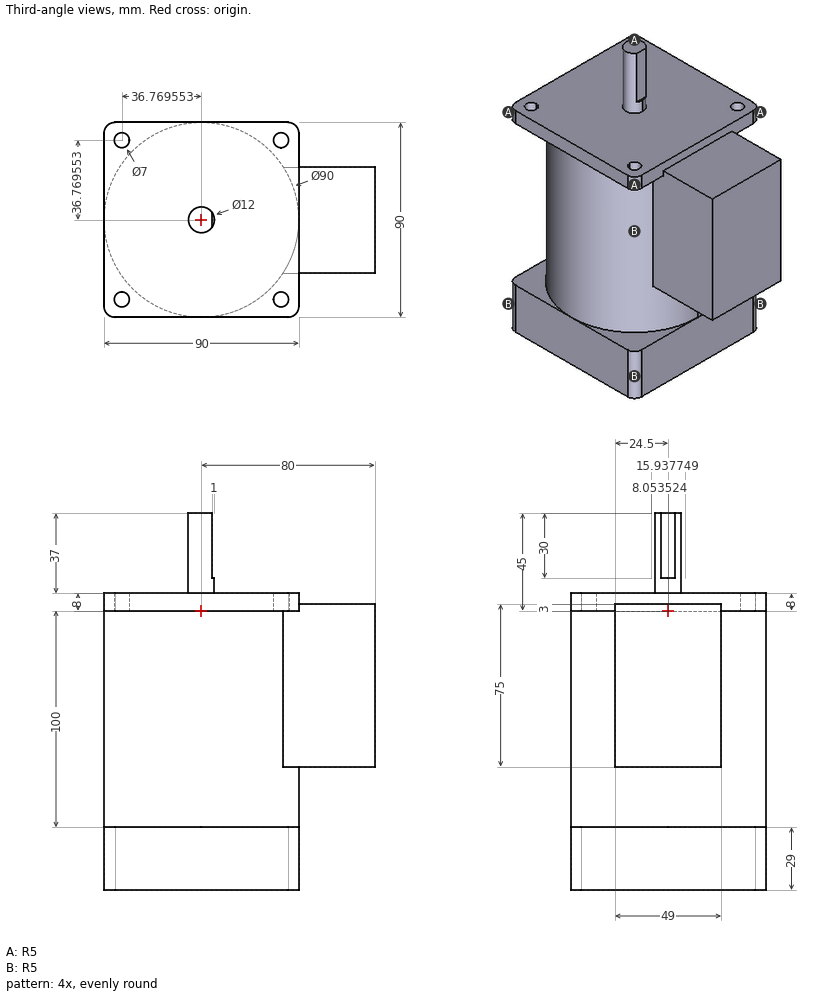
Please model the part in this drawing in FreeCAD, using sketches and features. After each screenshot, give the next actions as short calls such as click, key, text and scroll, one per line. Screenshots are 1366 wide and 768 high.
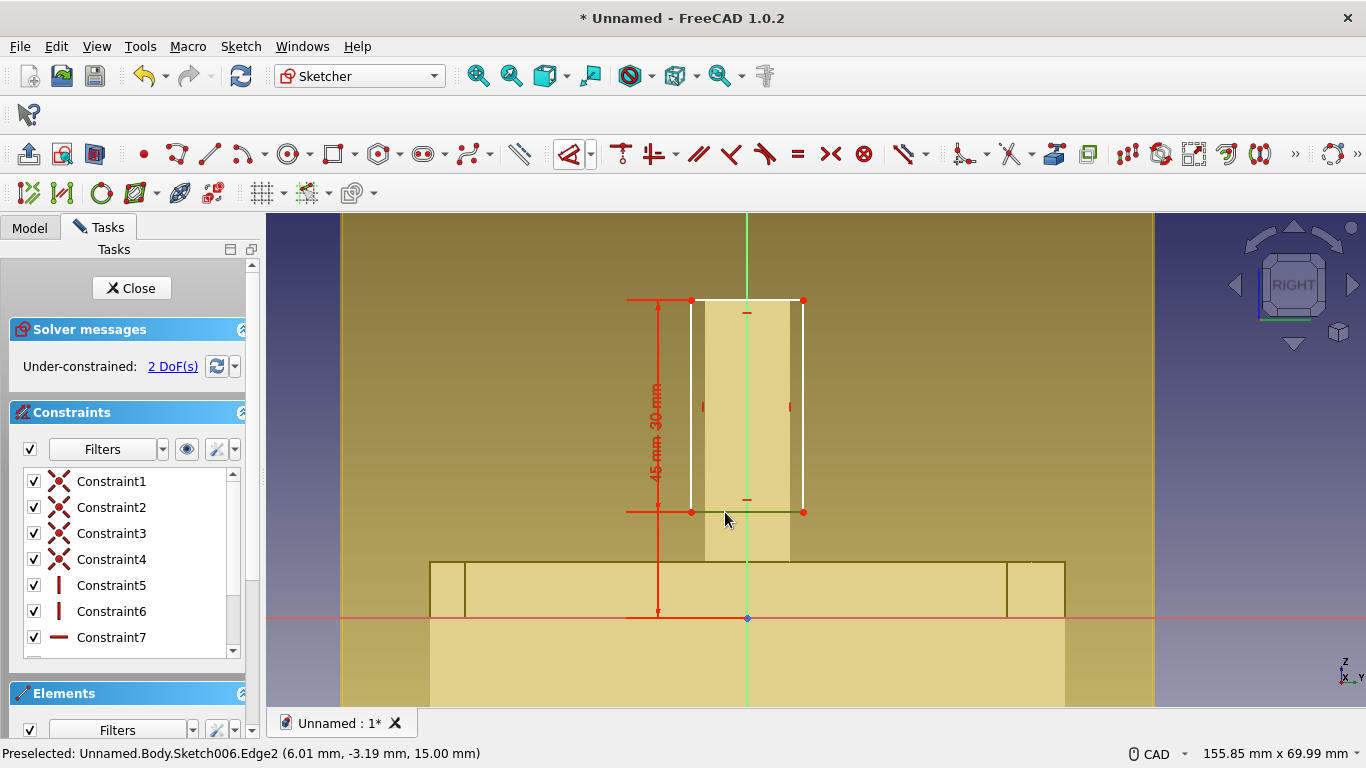
key(l)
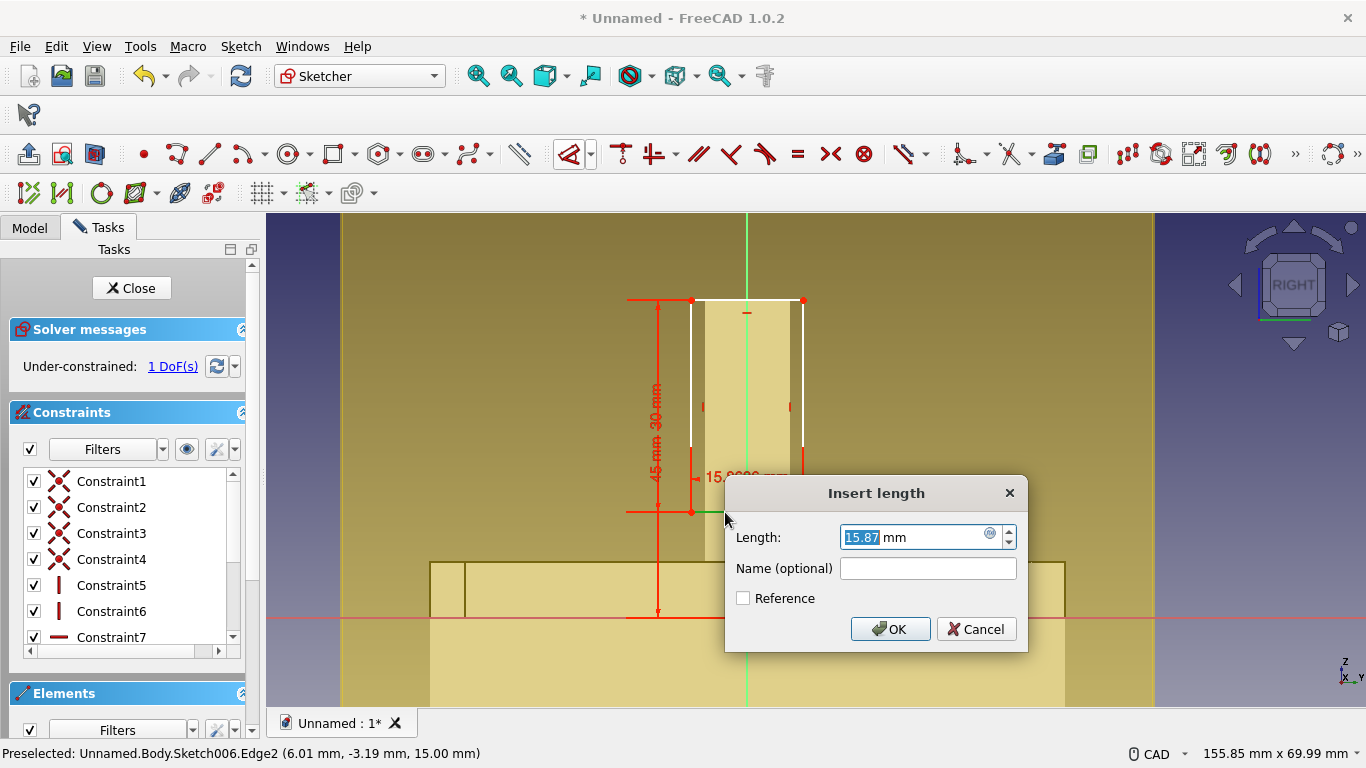
text(15.937749)
key(Return)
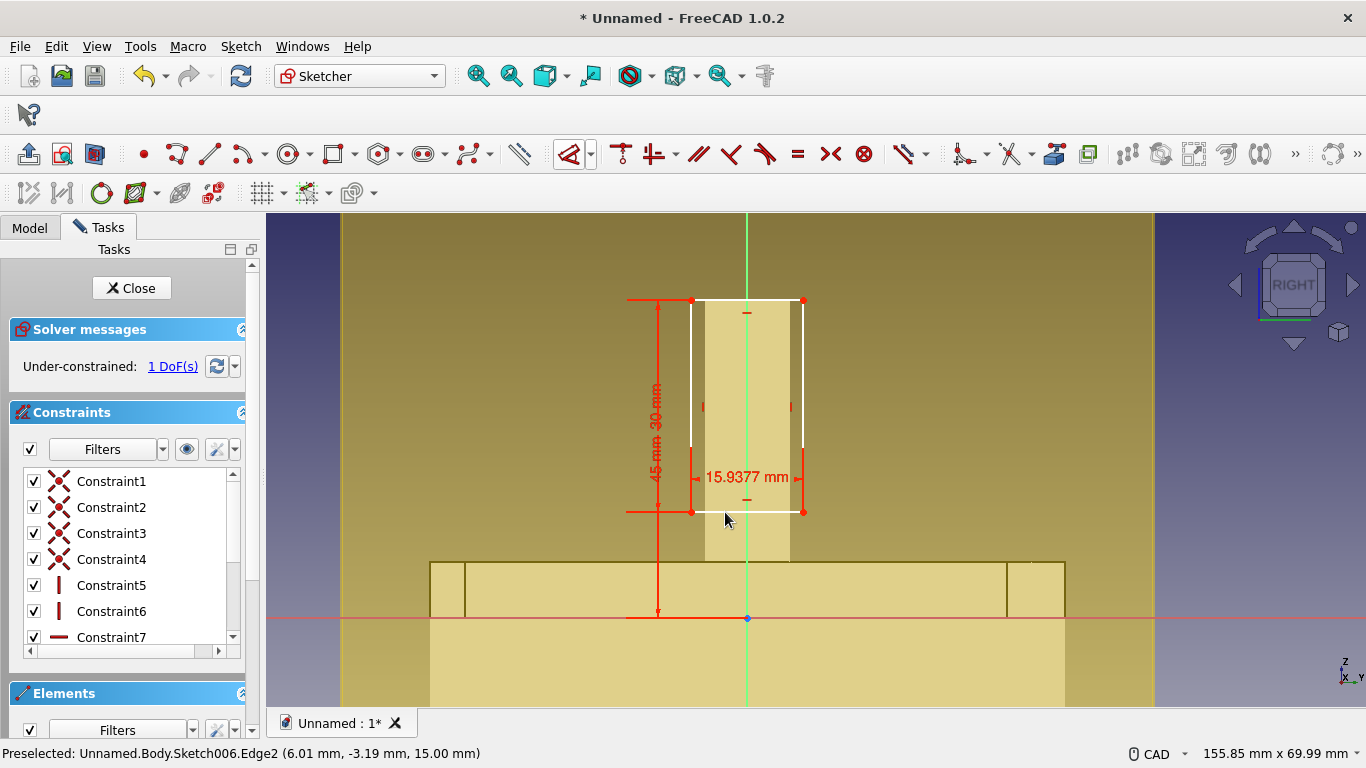
click(691, 300)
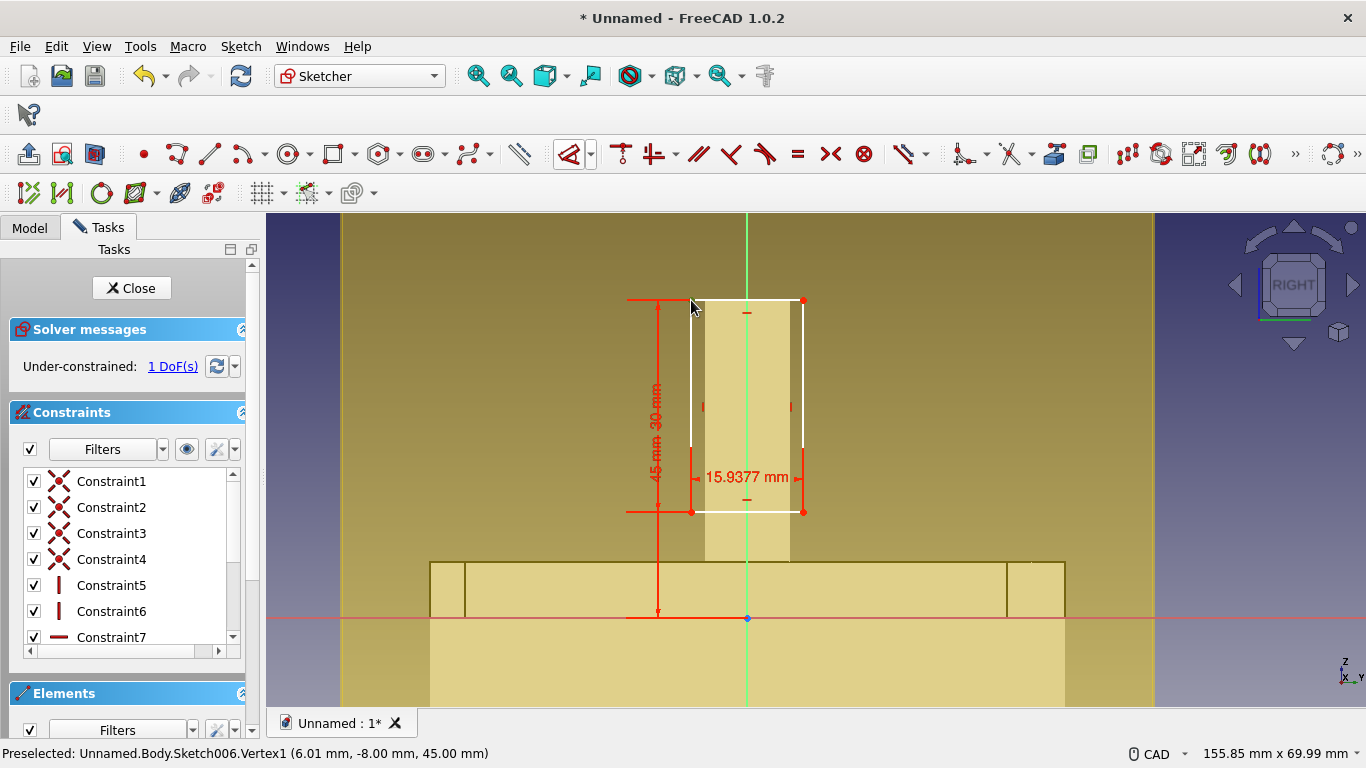
key(l)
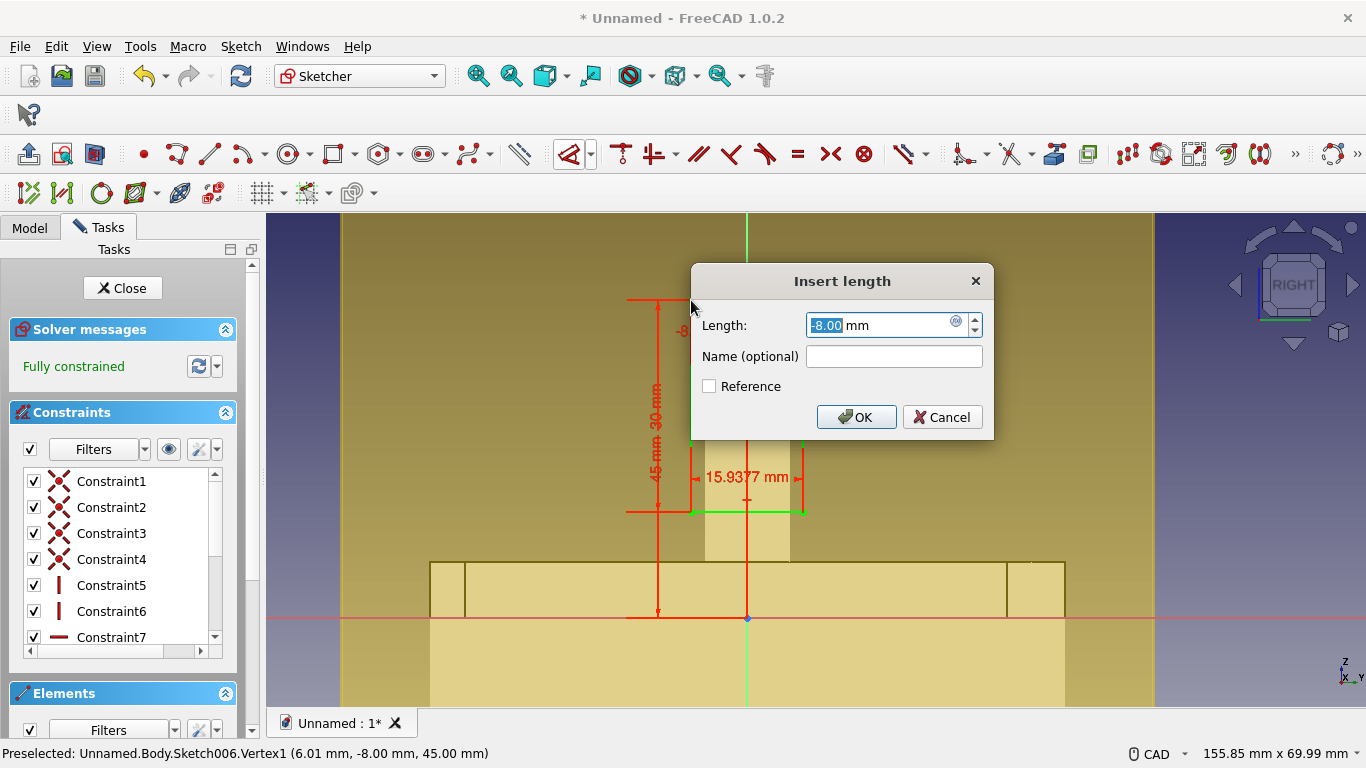
text(-8.053524)
key(Return)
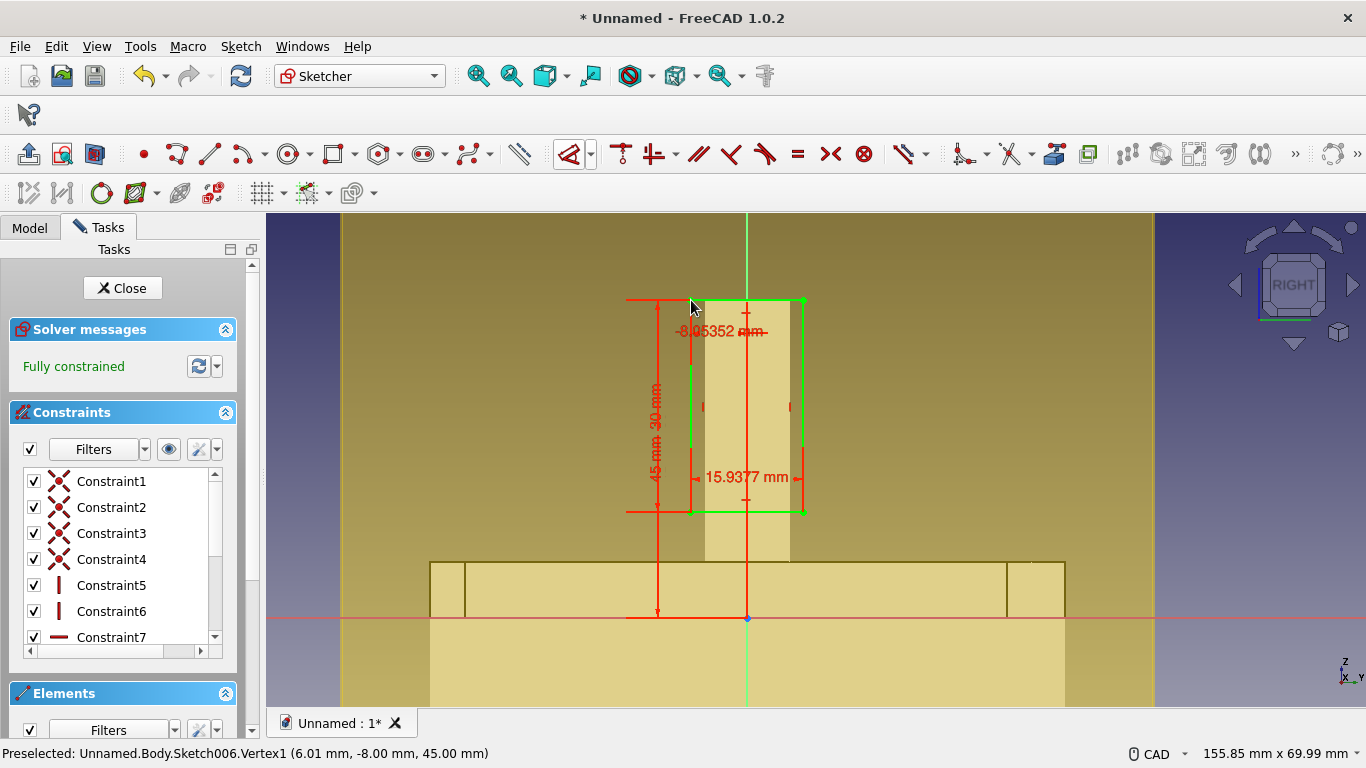
click(123, 288)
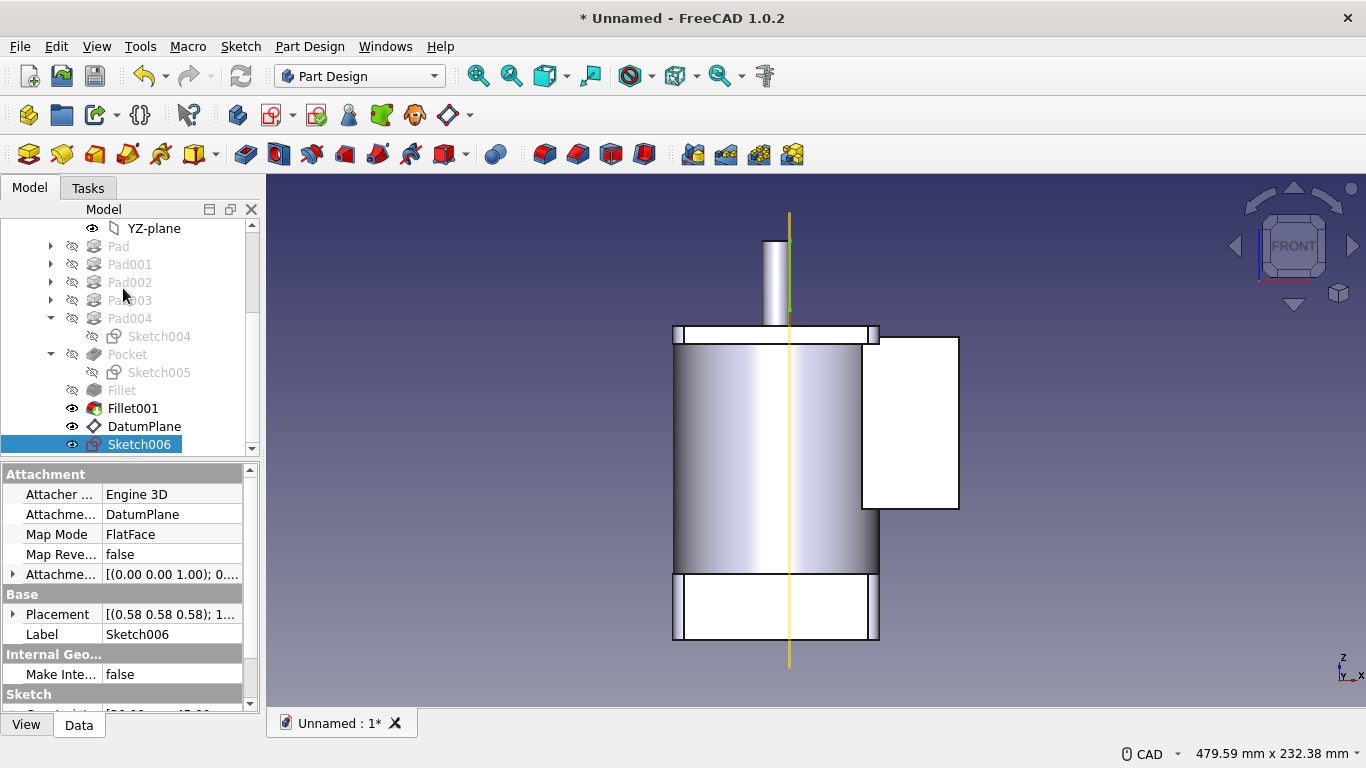
click(246, 154)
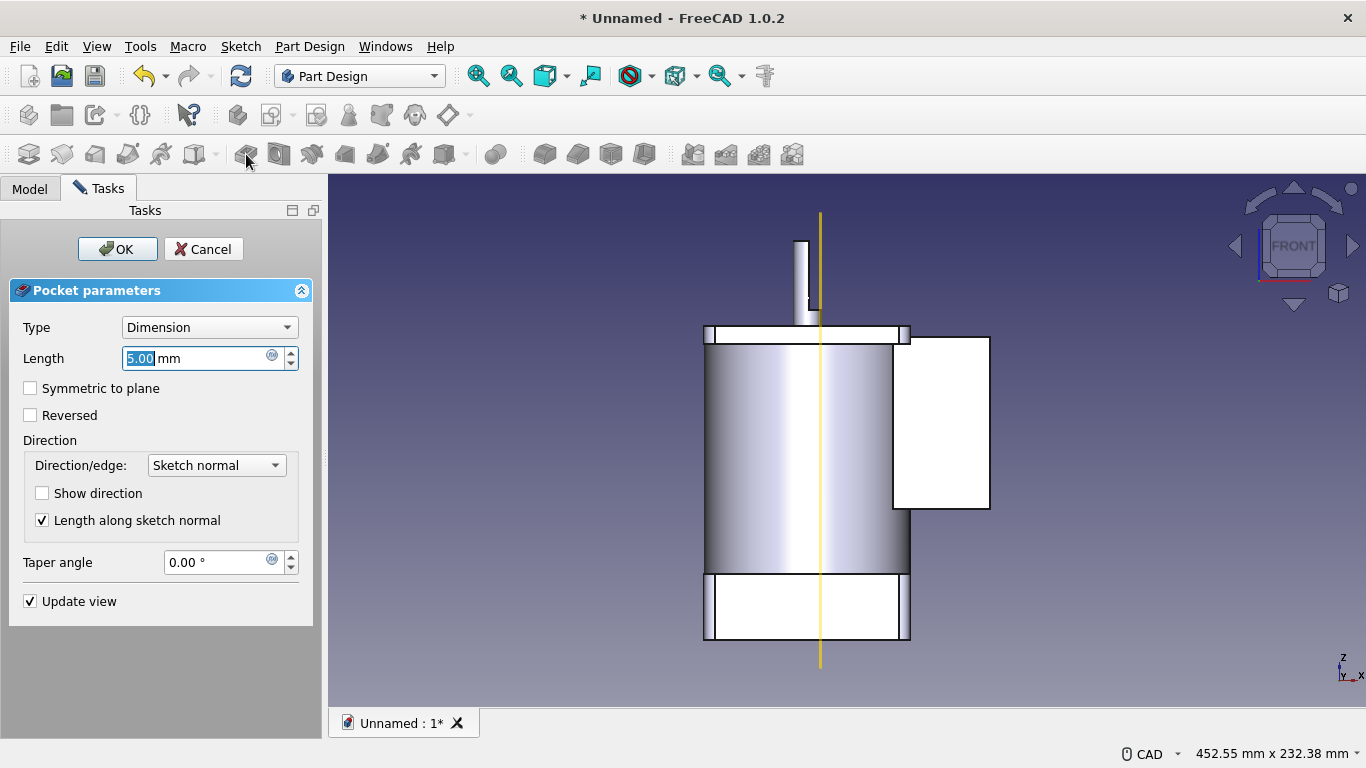
text(1)
key(Tab)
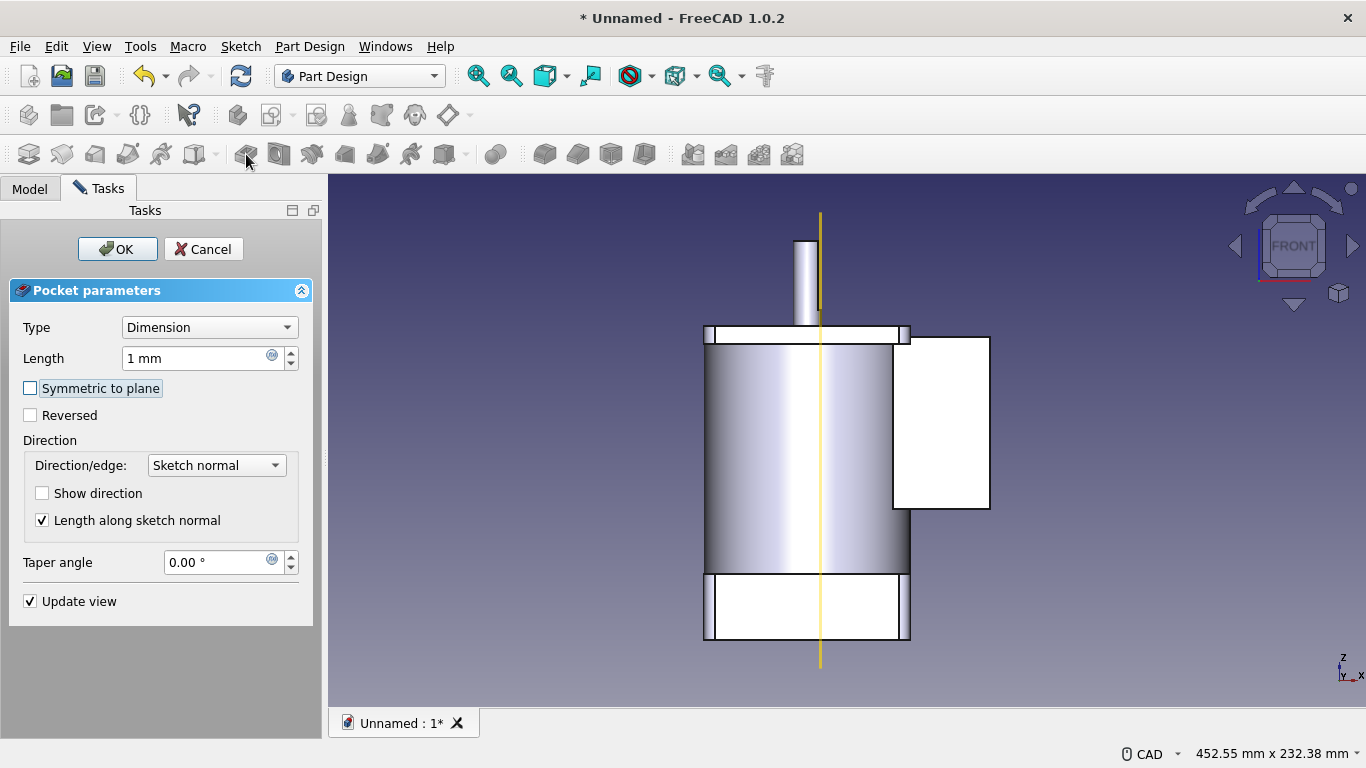
click(118, 249)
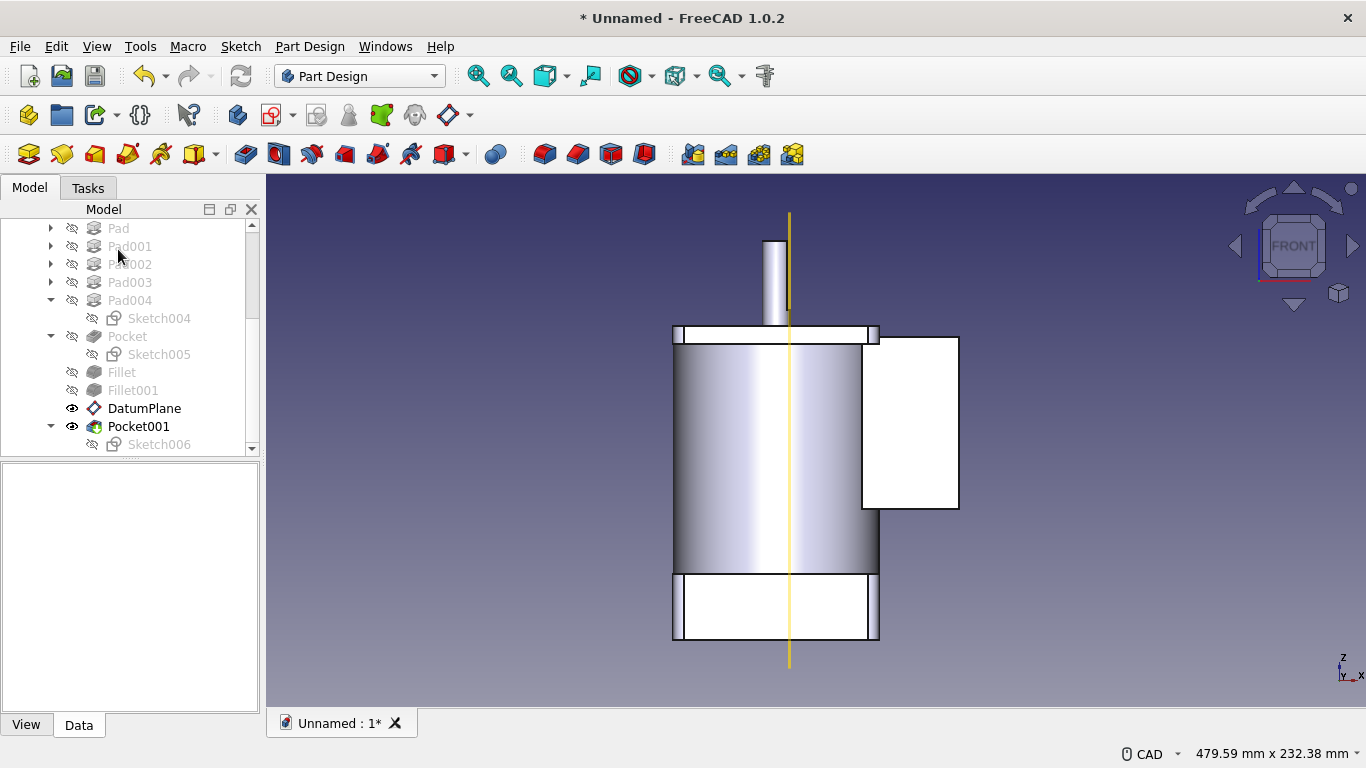
click(117, 408)
key(space)